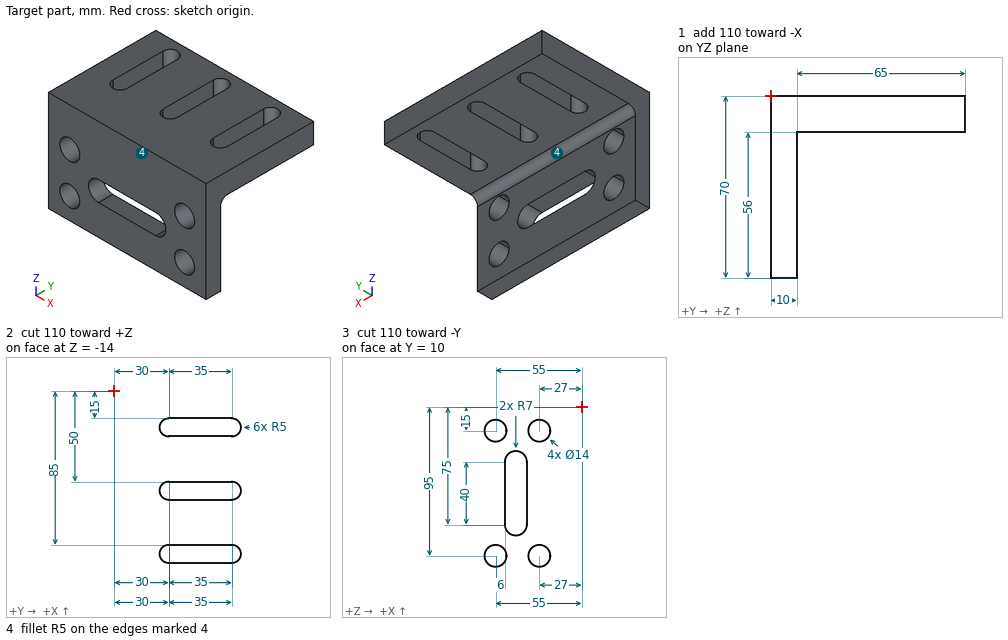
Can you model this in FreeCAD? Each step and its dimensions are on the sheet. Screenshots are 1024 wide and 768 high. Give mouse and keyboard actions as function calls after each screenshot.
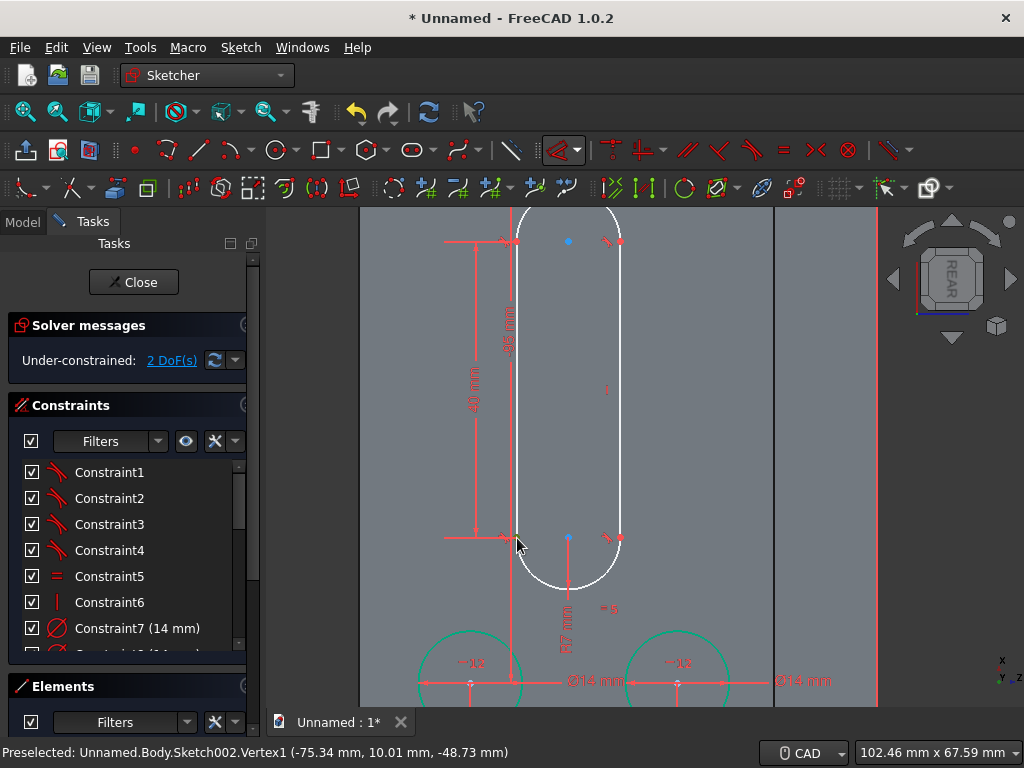
scroll(518, 538, down, 4)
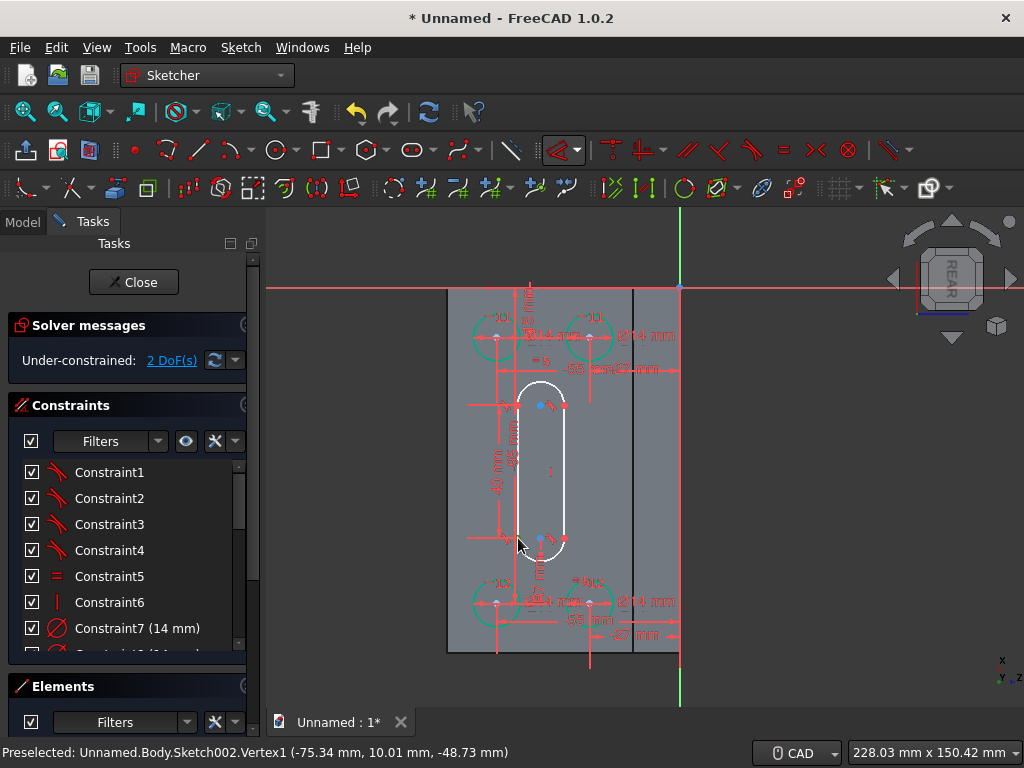
scroll(497, 604, up, 4)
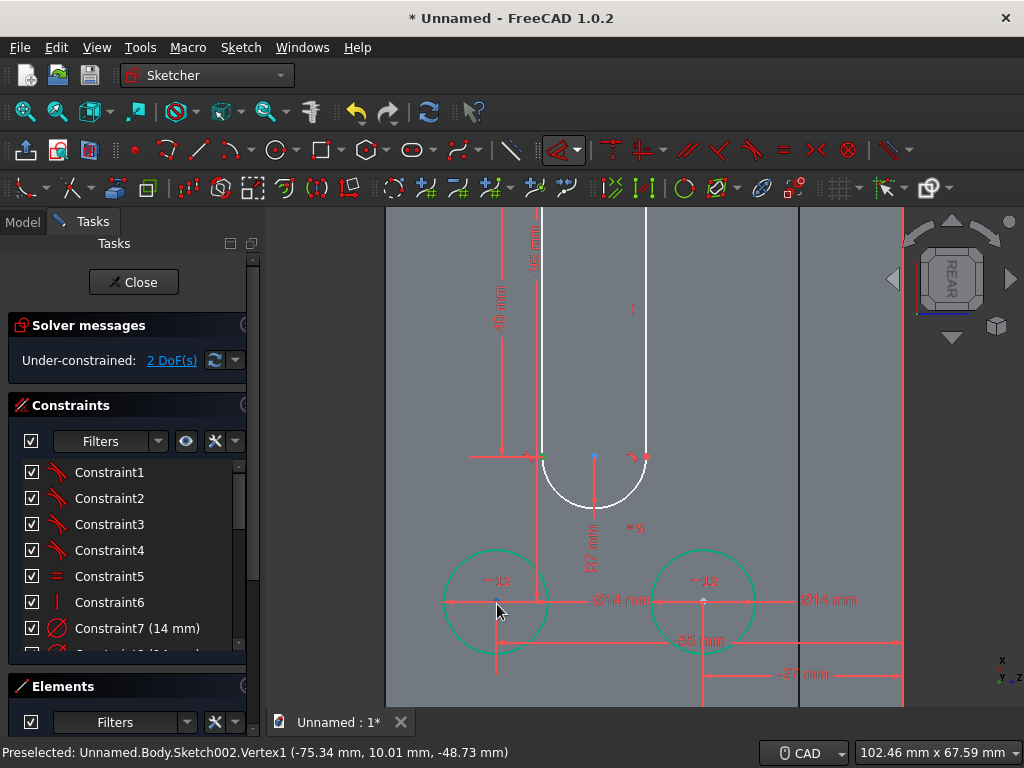
click(496, 602)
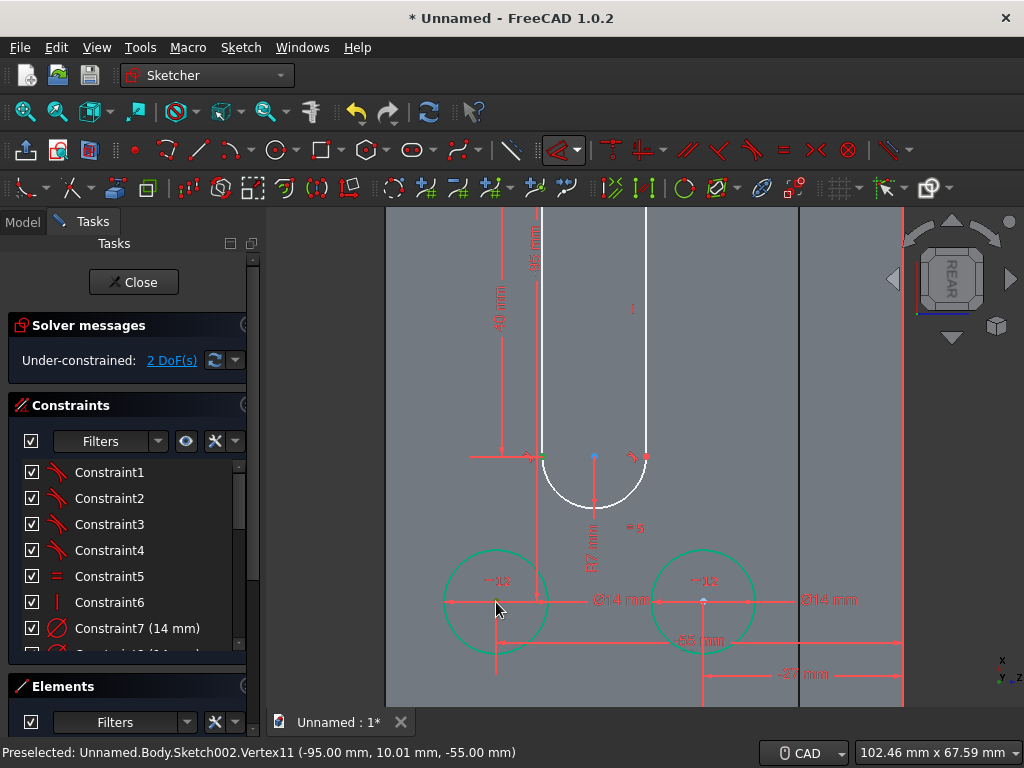
click(580, 150)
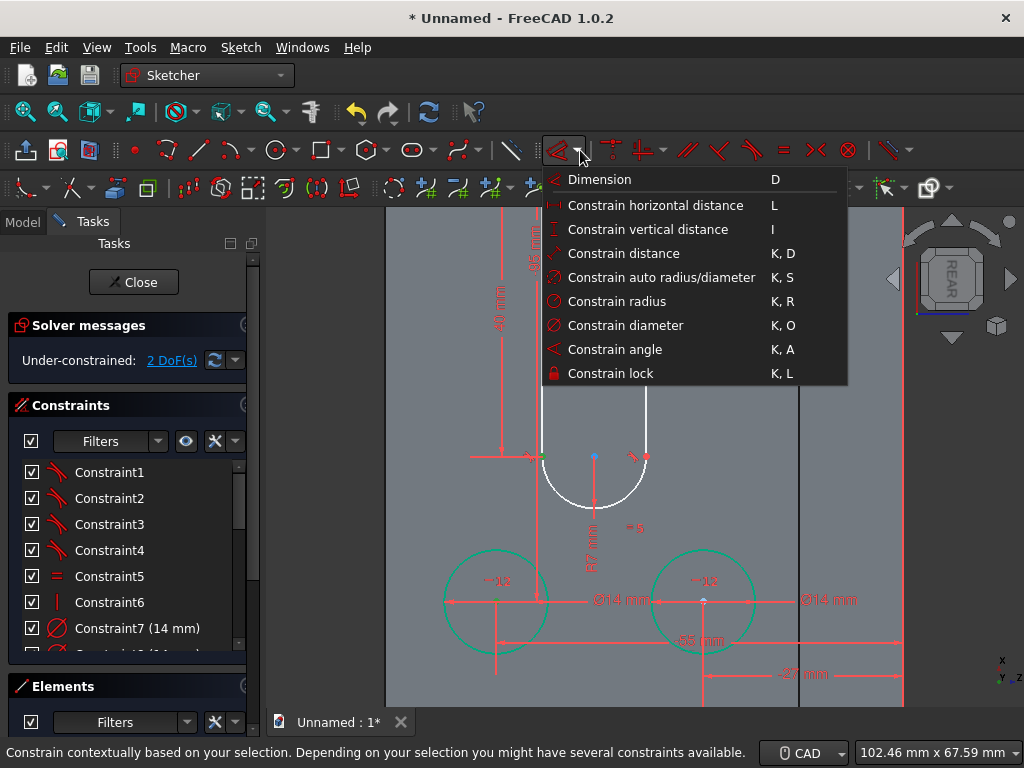
click(695, 205)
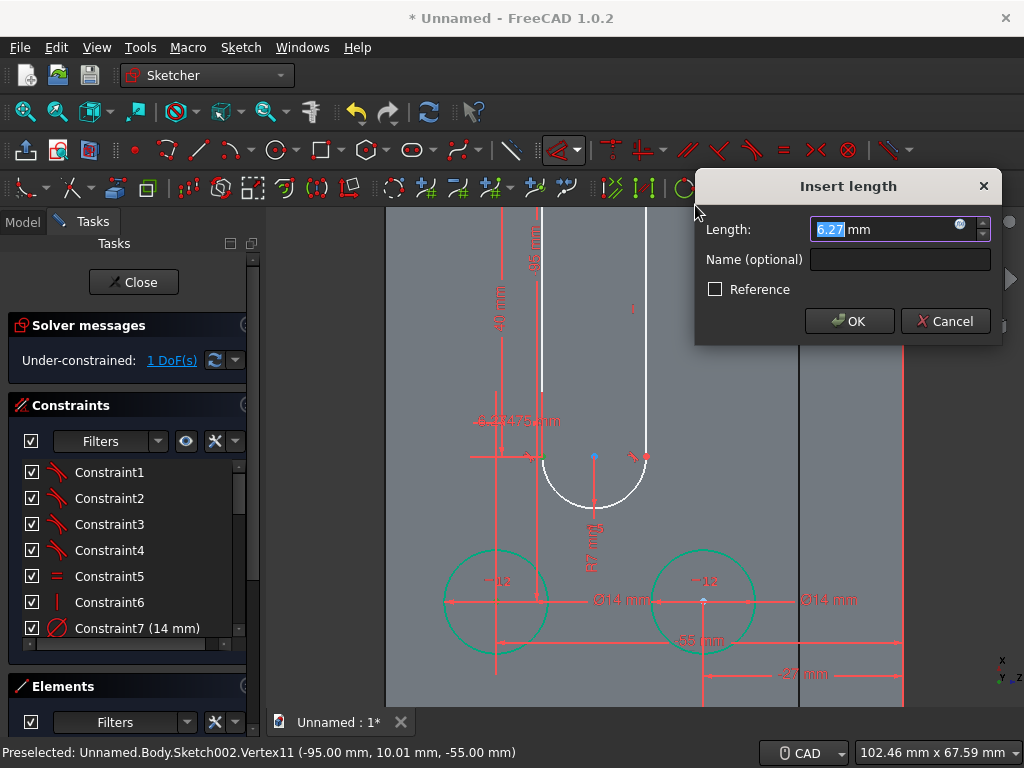
text(6)
key(Return)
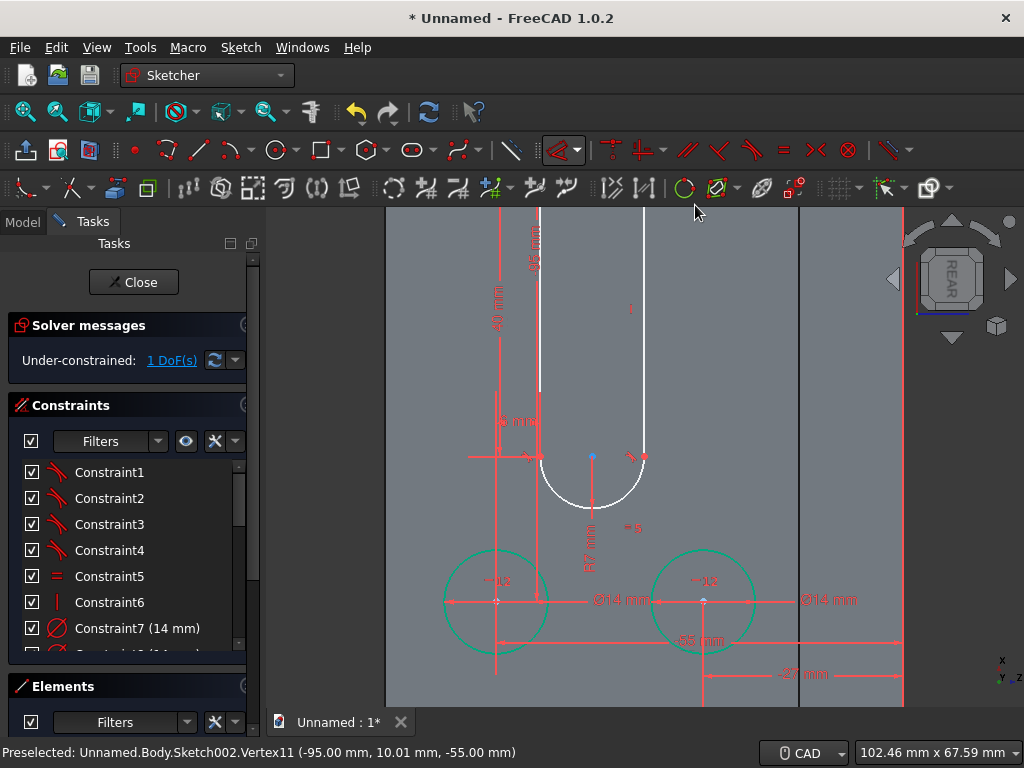
click(540, 457)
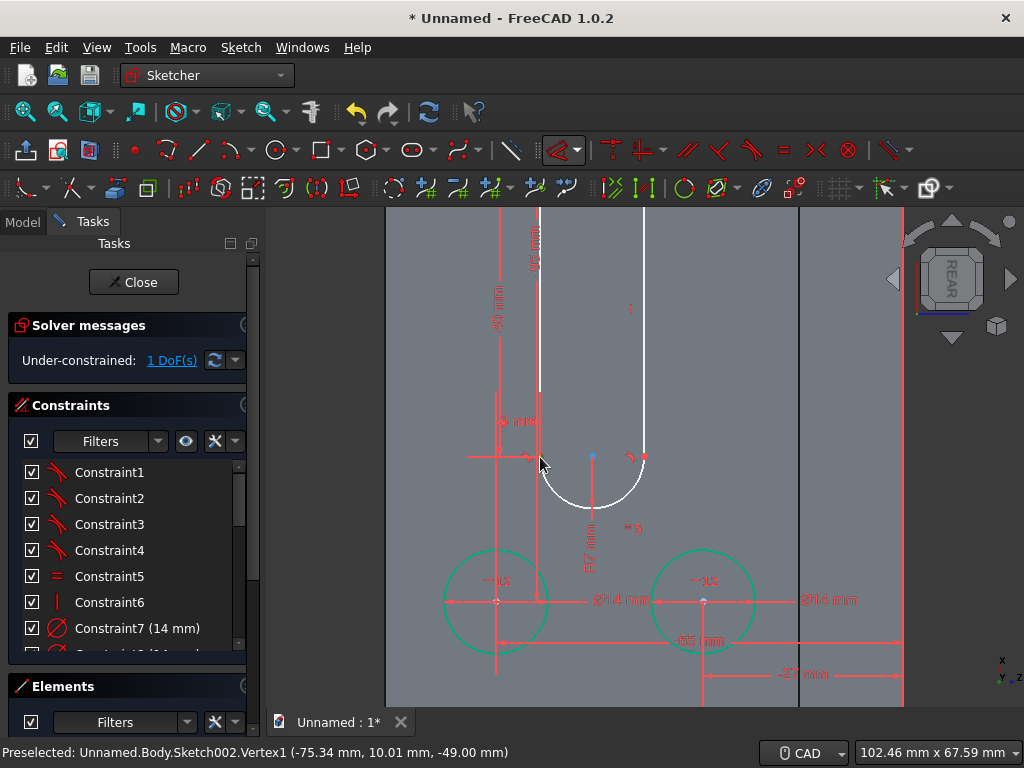
click(580, 150)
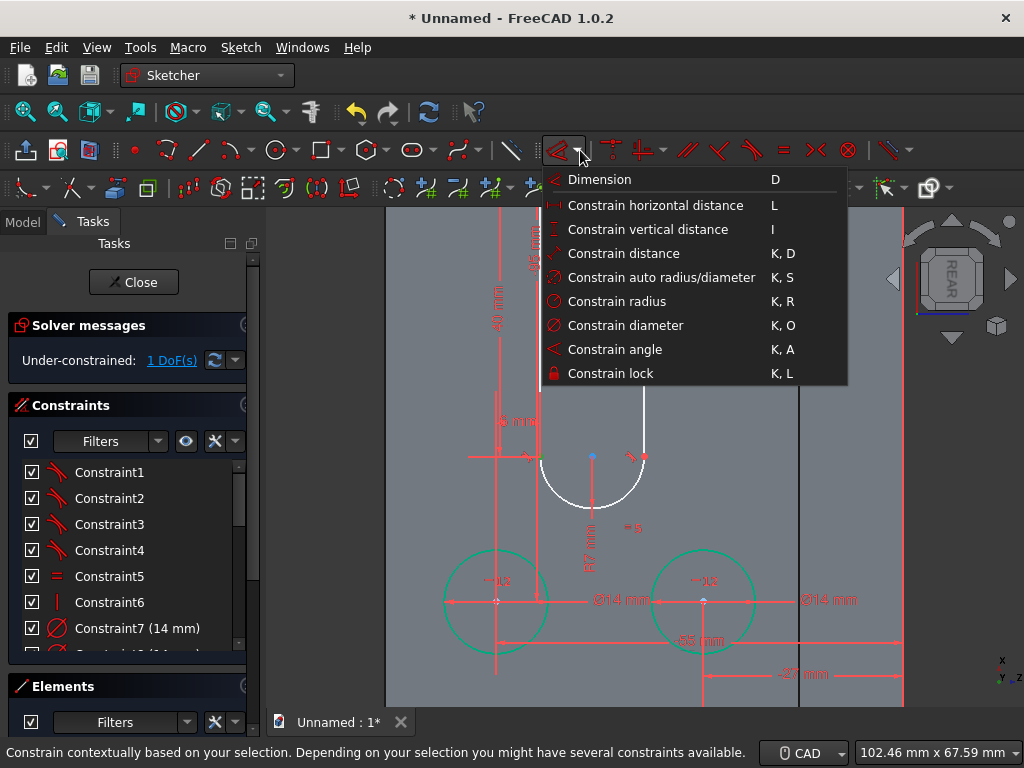
click(695, 229)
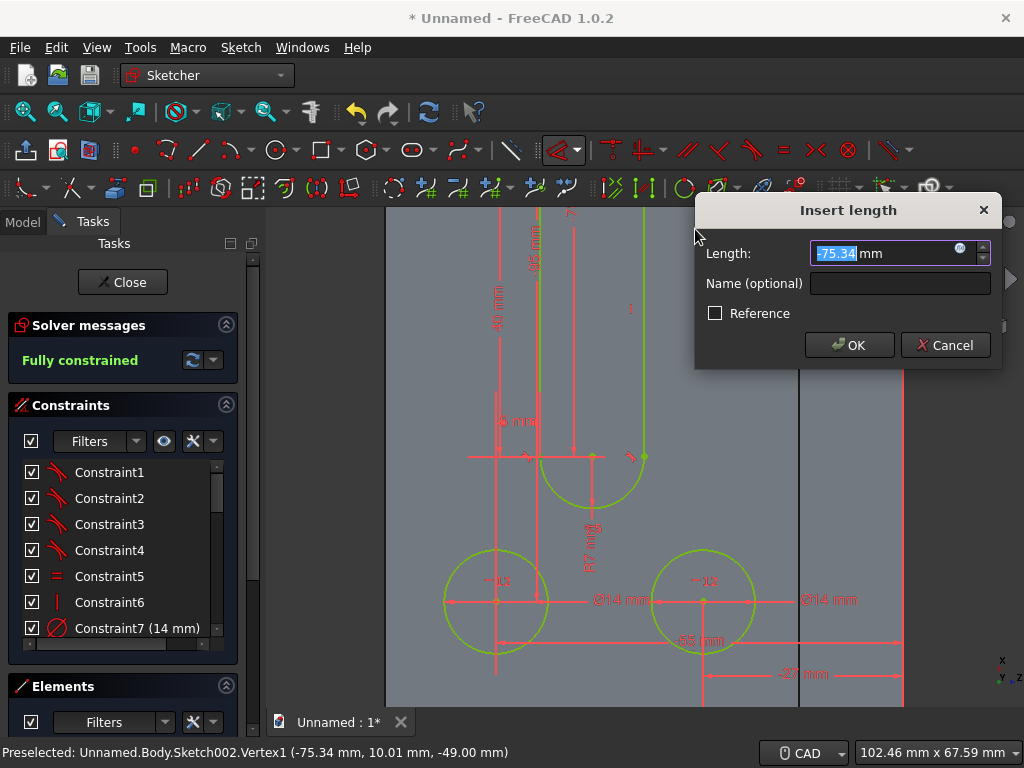
text(-75)
key(Return)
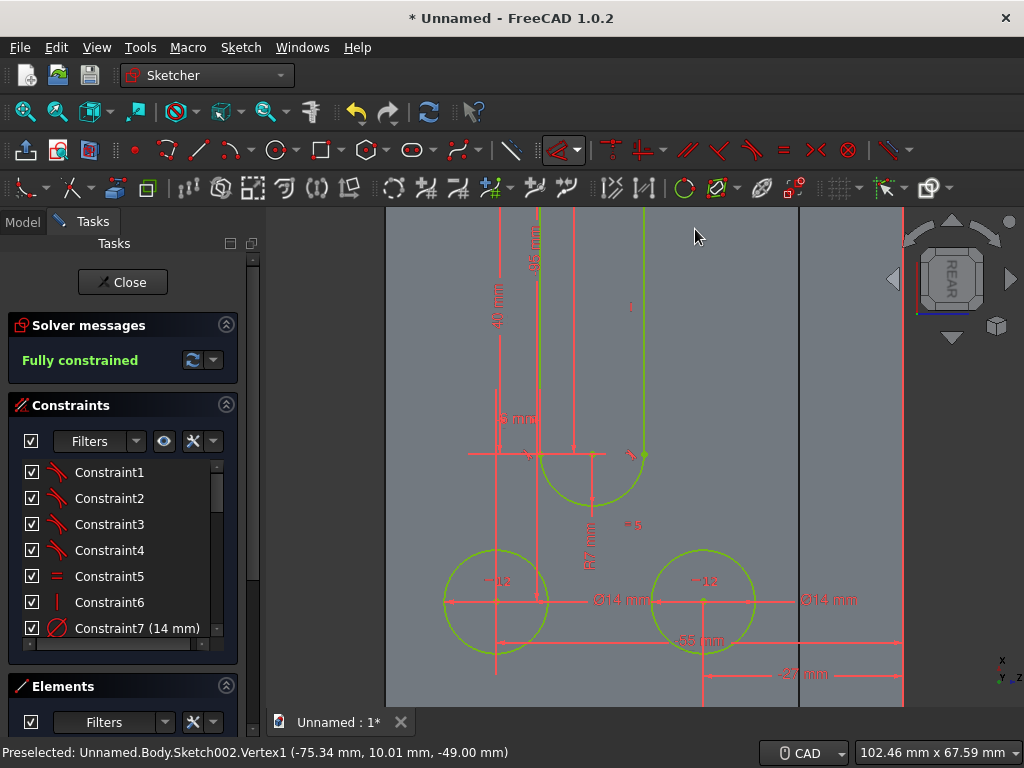
click(123, 282)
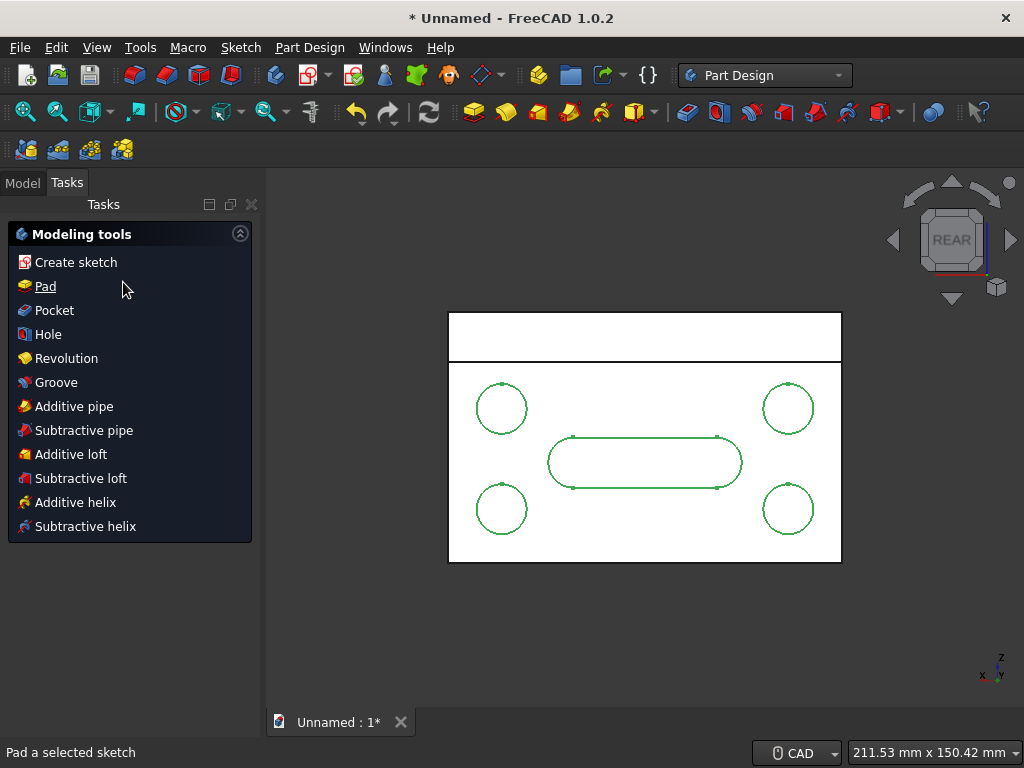
click(688, 112)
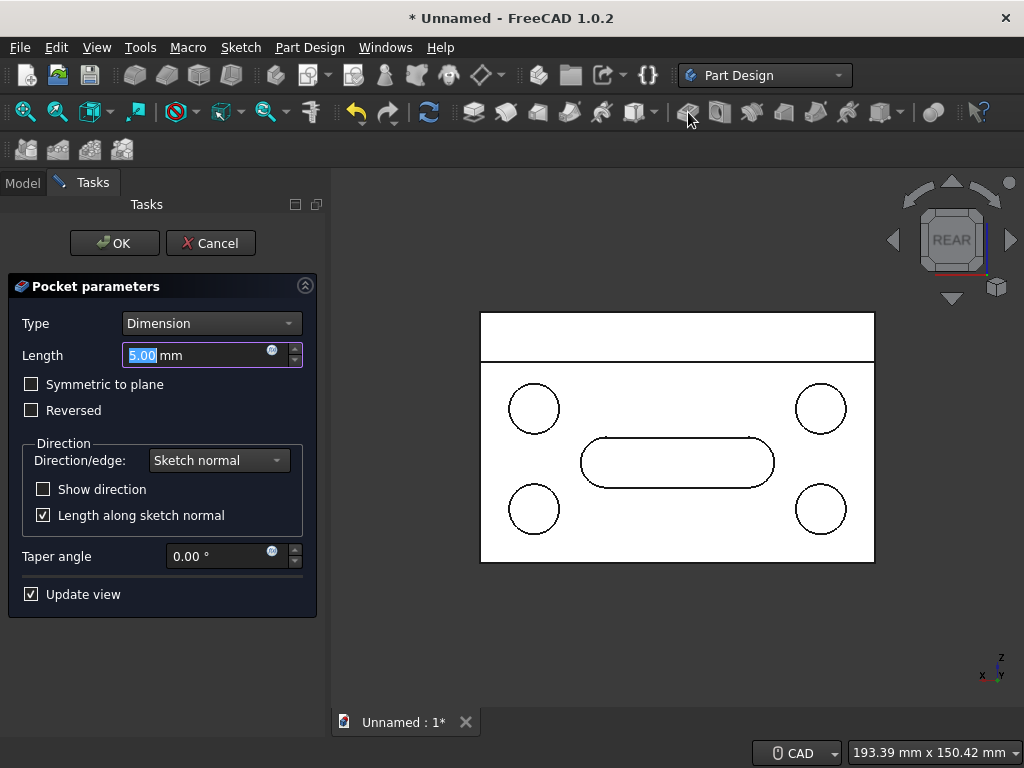
text(110)
key(Tab)